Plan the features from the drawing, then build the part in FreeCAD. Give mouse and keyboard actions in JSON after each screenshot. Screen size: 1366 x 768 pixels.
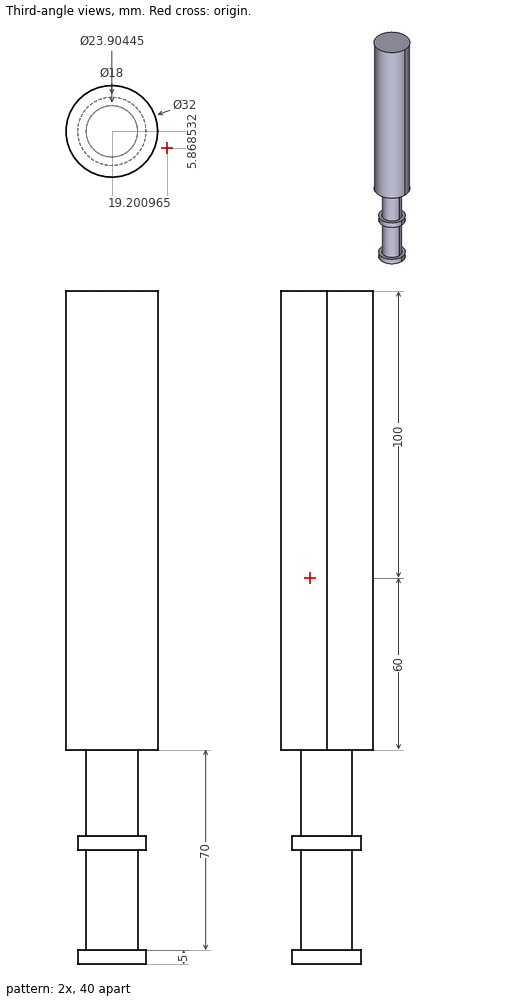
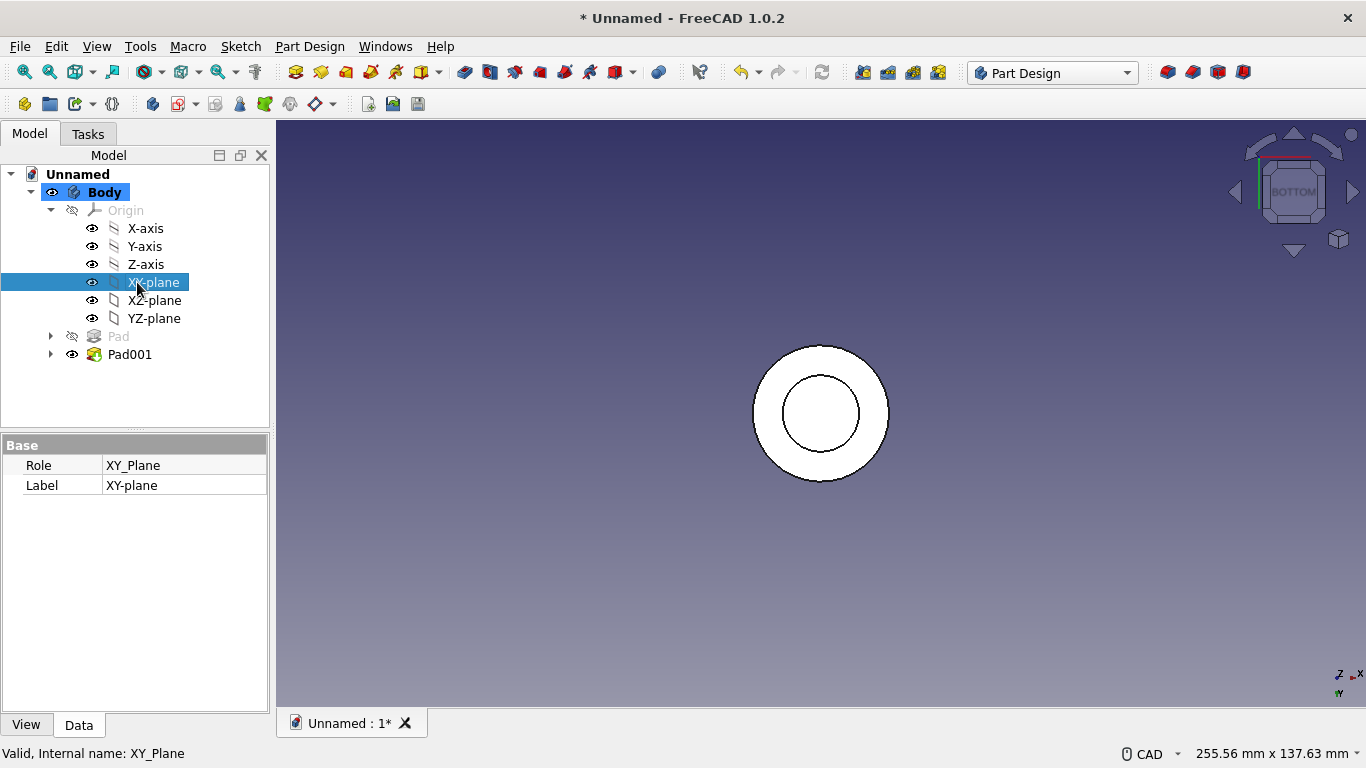
{"action": "left_click", "coordinate": [314, 104]}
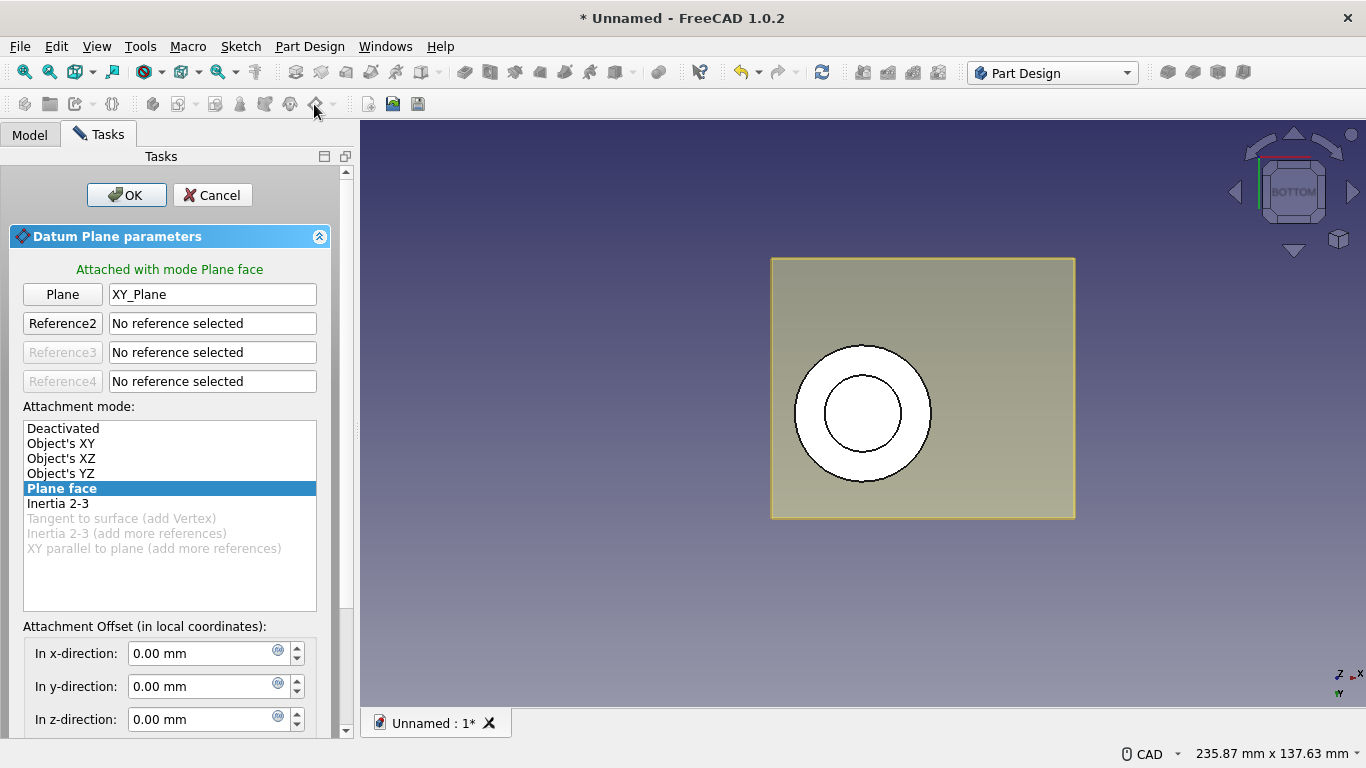
{"action": "triple_click", "coordinate": [210, 720]}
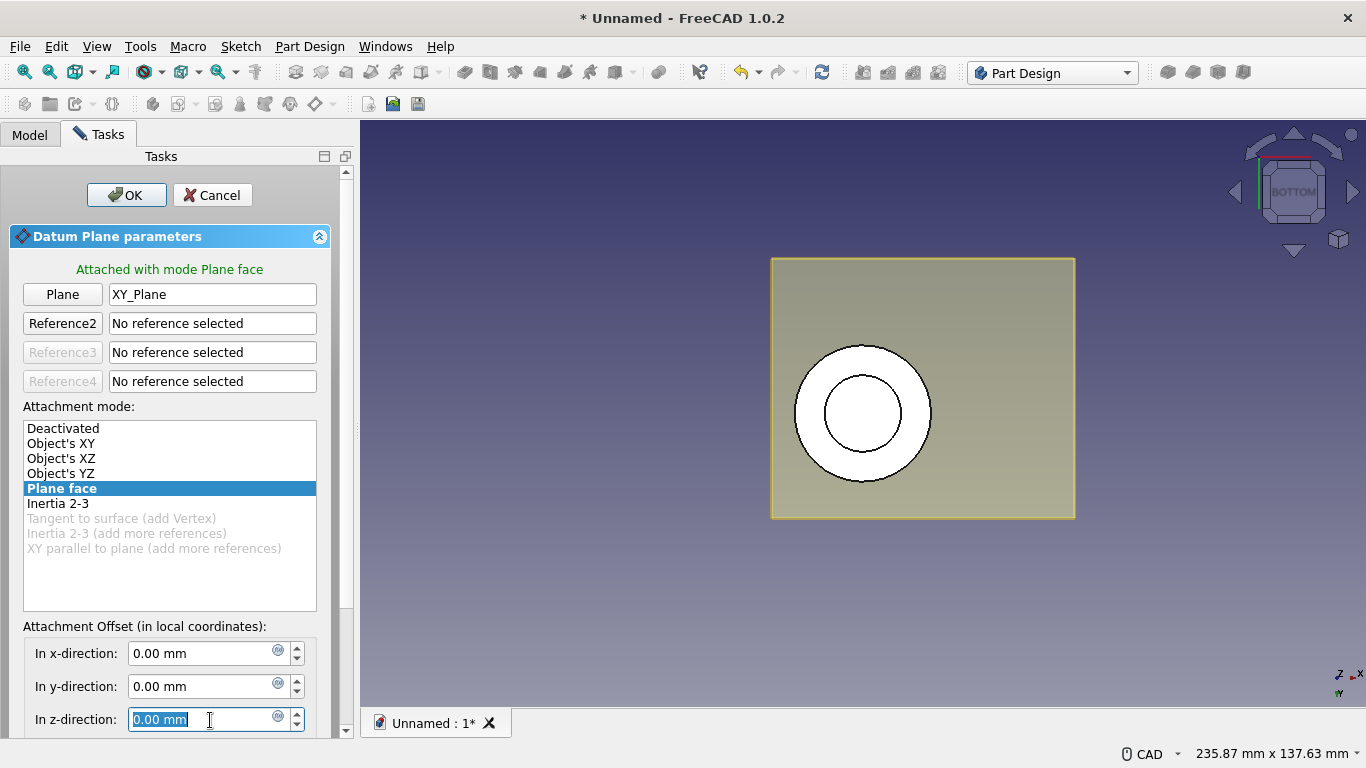
{"action": "type", "text": "100"}
{"action": "key", "text": "Tab"}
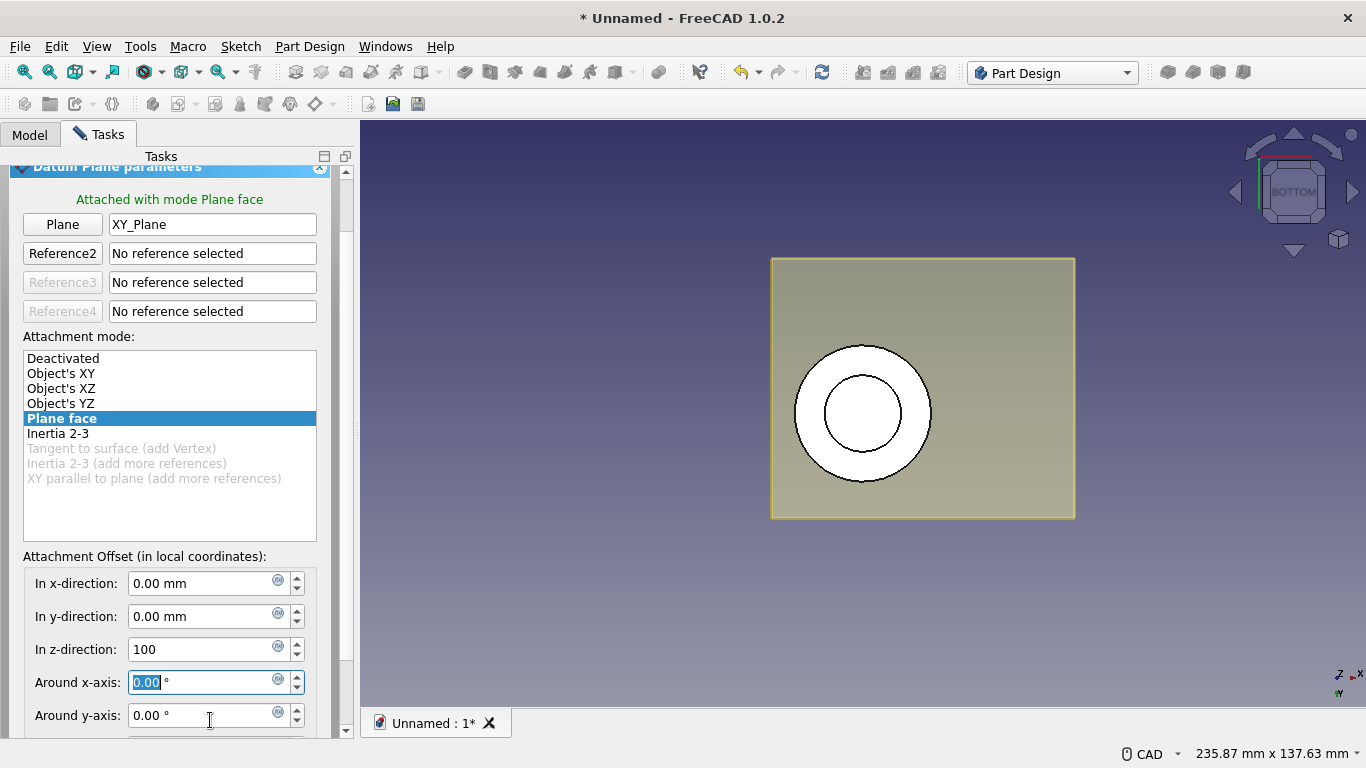
{"action": "scroll", "coordinate": [346, 452], "scroll_direction": "up", "scroll_amount": 2}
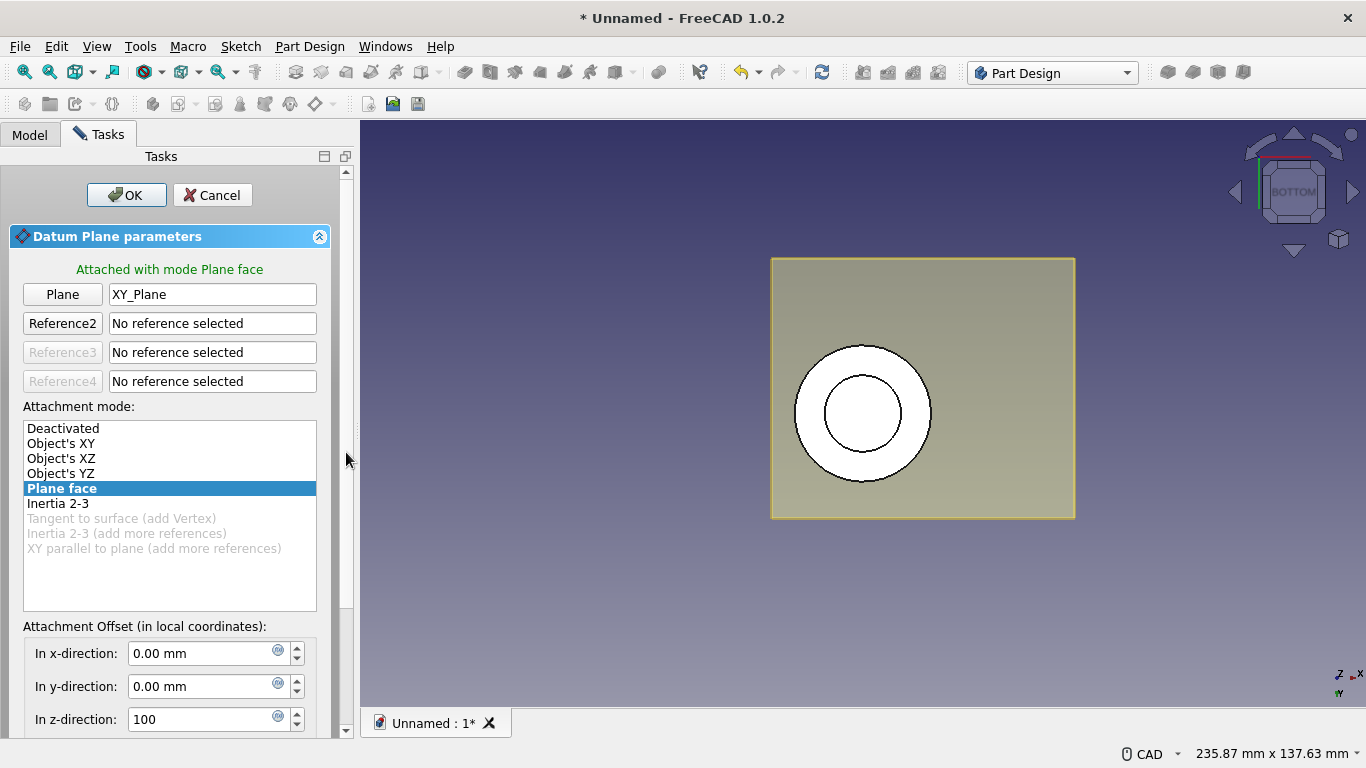
{"action": "left_click", "coordinate": [127, 195]}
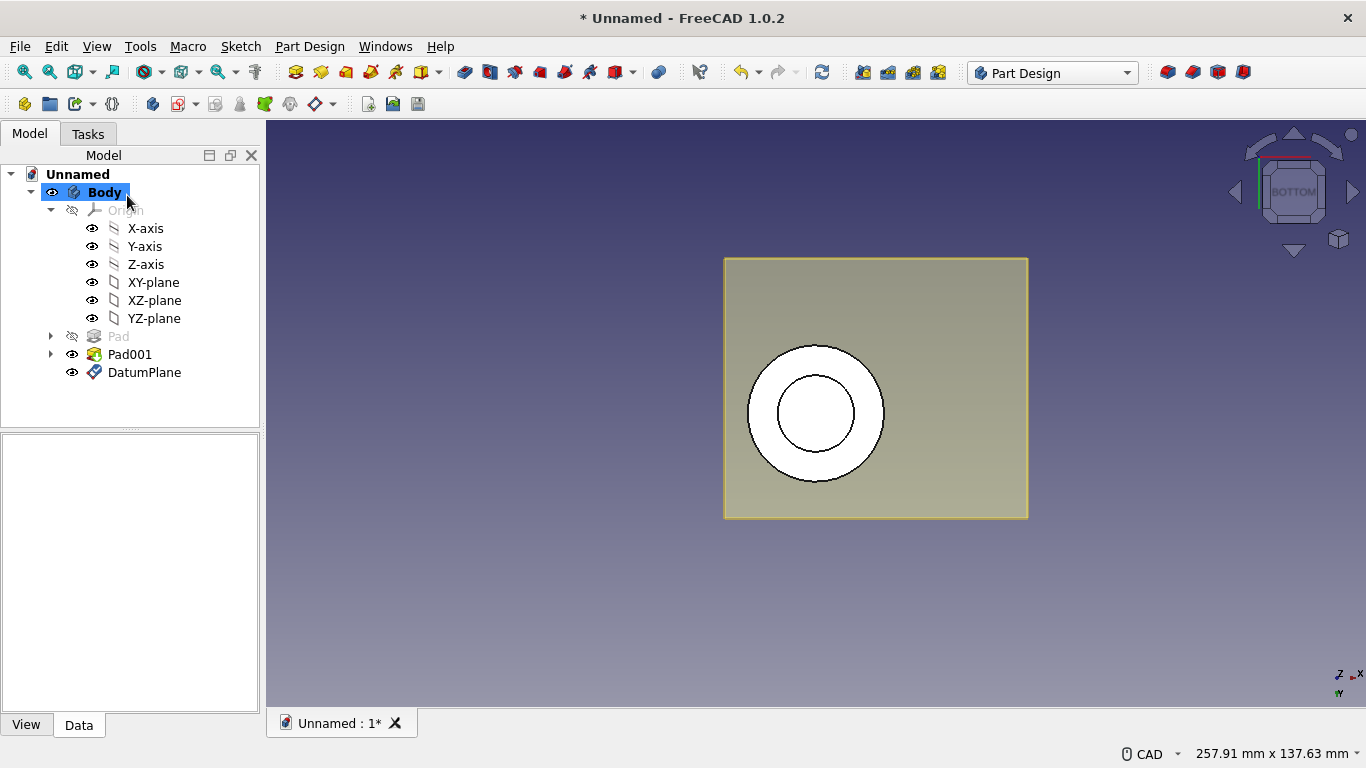
{"action": "left_click", "coordinate": [117, 372]}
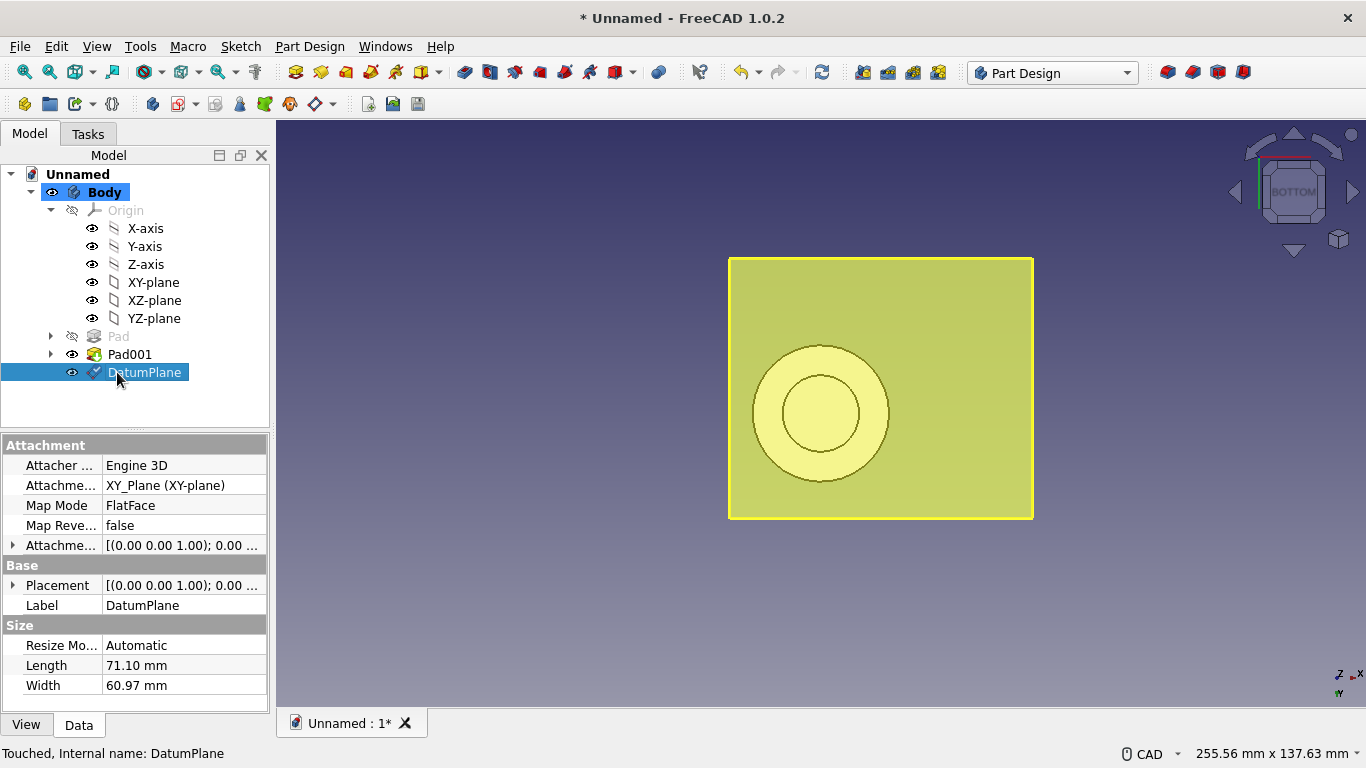
{"action": "left_click", "coordinate": [178, 104]}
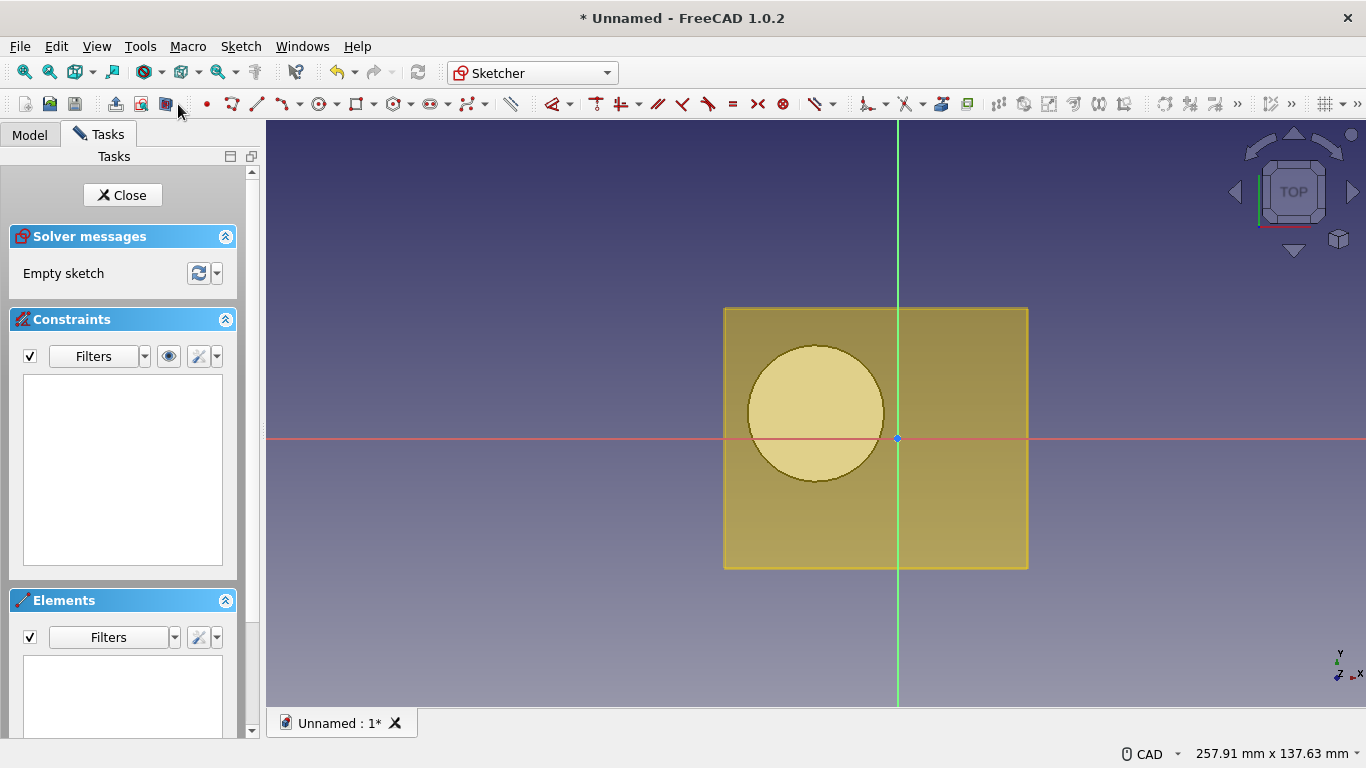
{"action": "scroll", "coordinate": [866, 413], "scroll_direction": "up", "scroll_amount": 5}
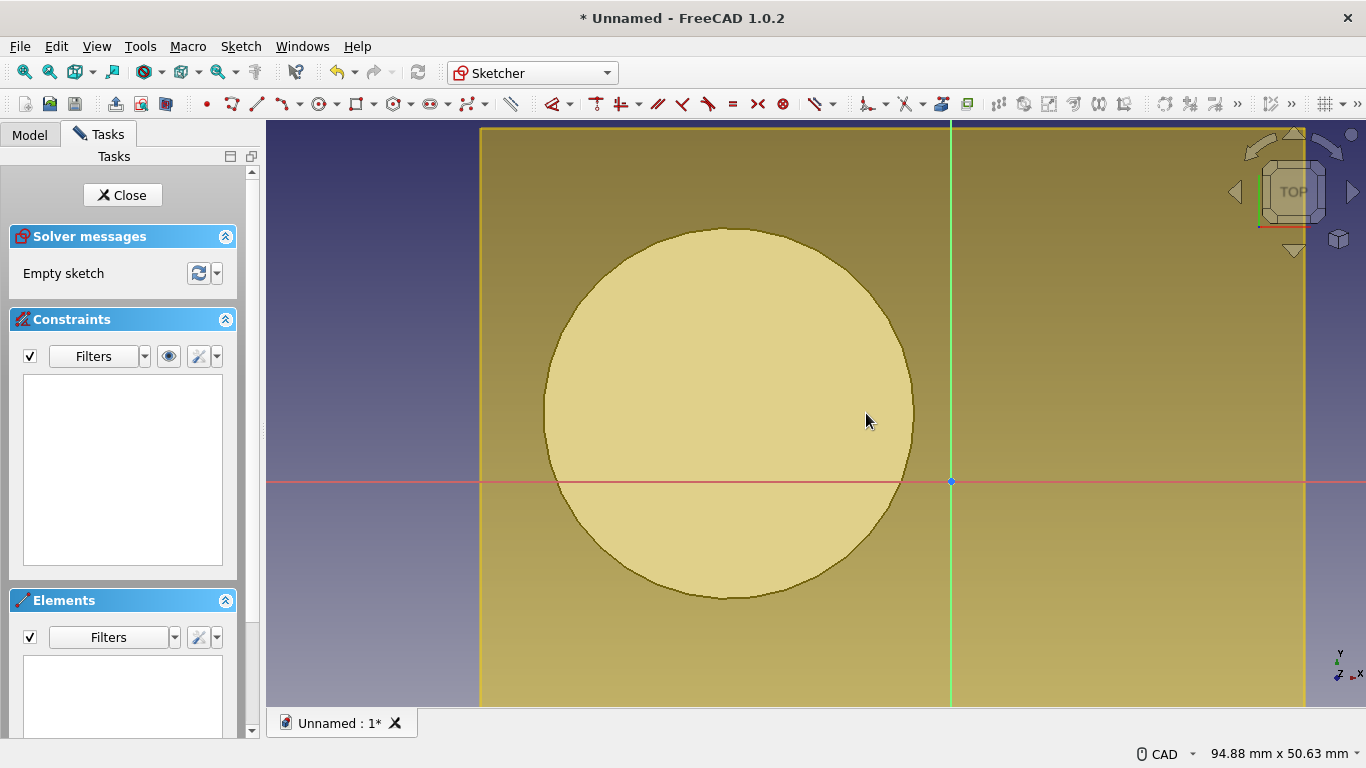
{"action": "key", "text": "g c"}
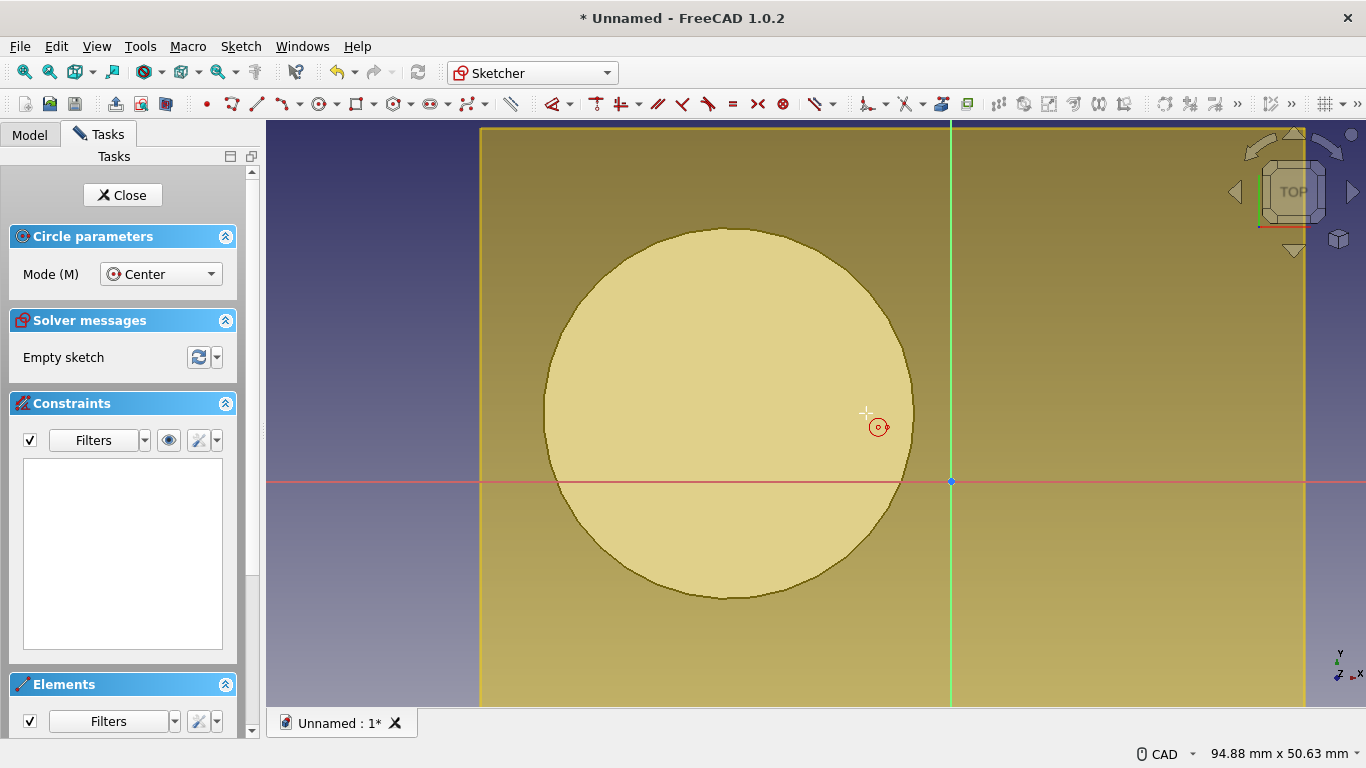
{"action": "left_click", "coordinate": [729, 413]}
{"action": "mouse_move", "coordinate": [860, 282]}